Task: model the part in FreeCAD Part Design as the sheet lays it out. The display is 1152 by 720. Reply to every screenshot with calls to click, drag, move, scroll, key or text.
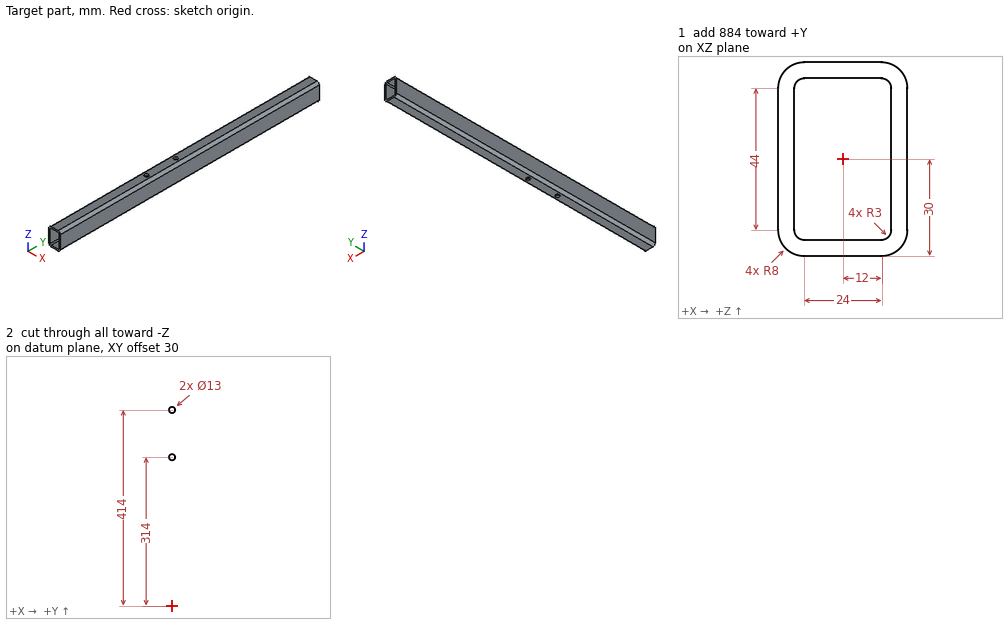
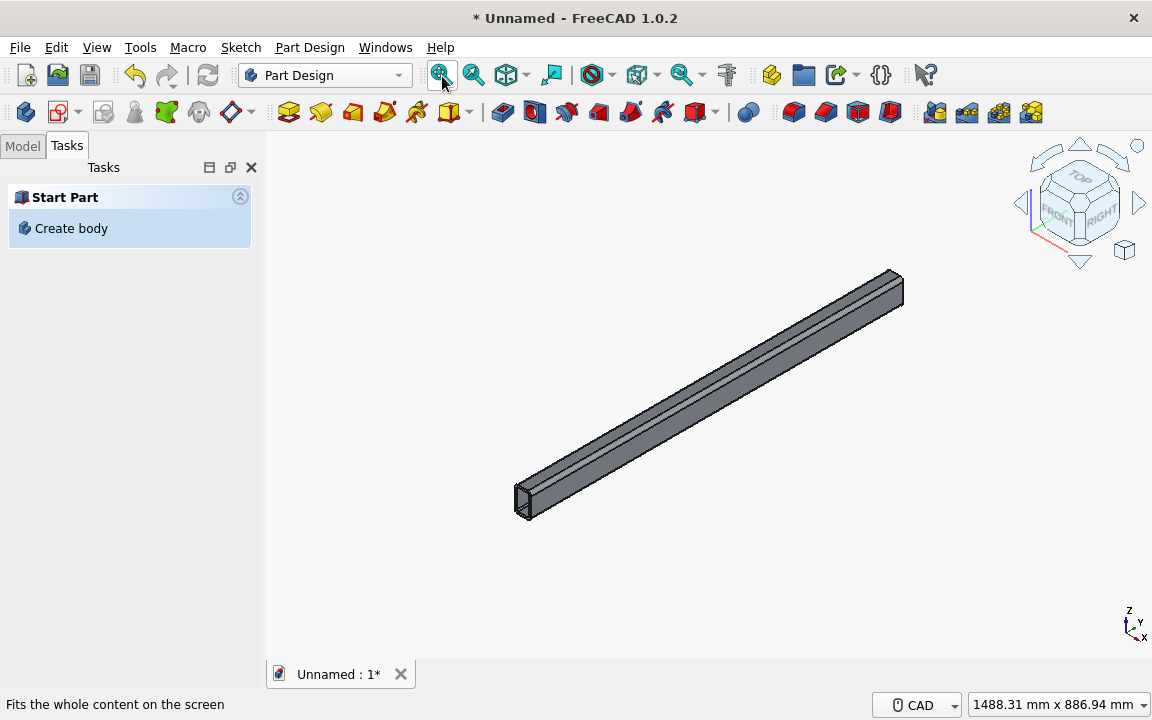
key(2)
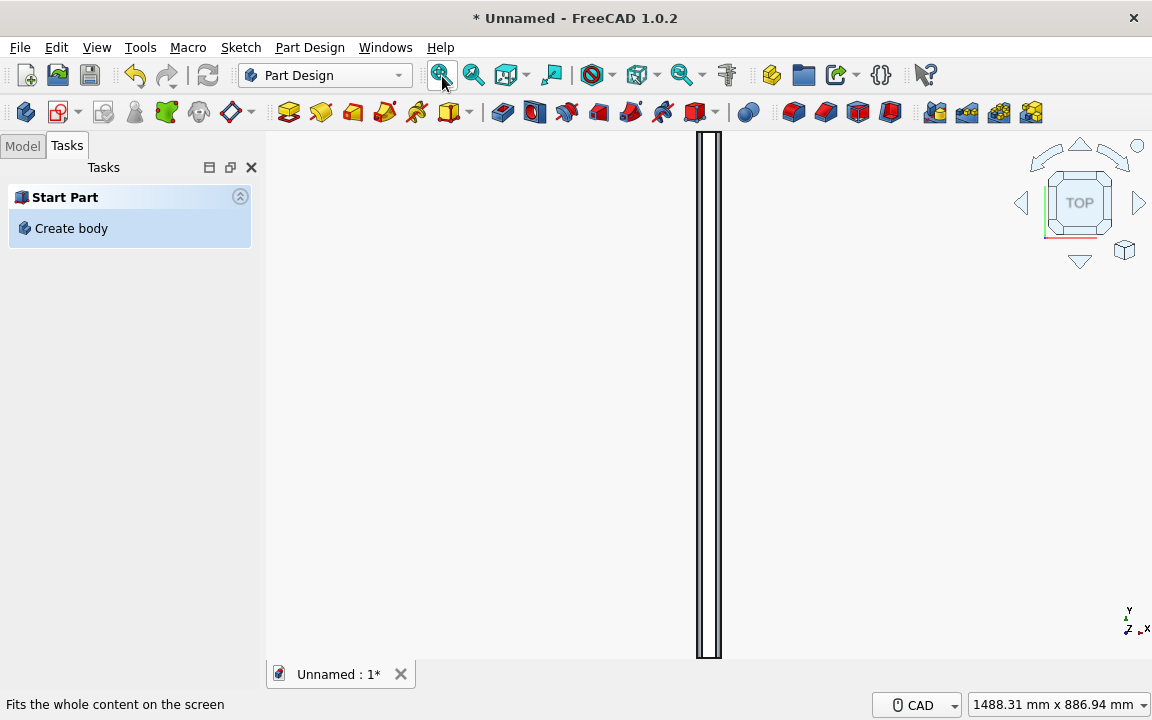
key(4)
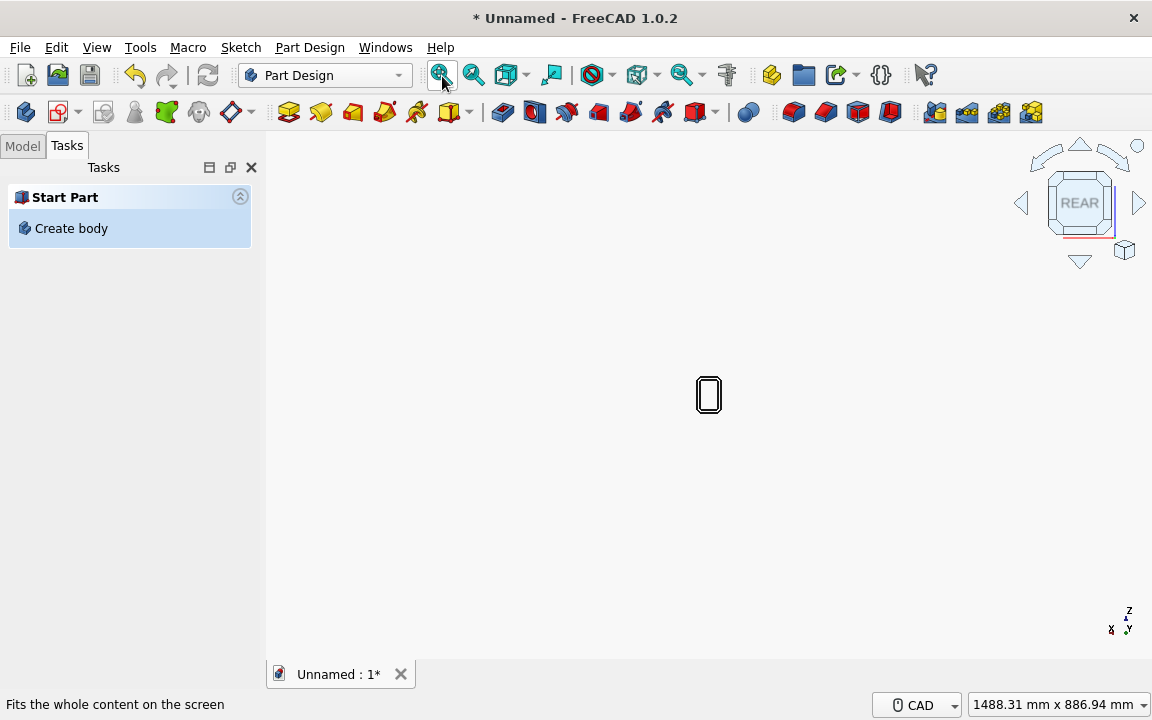
key(v)
key(f)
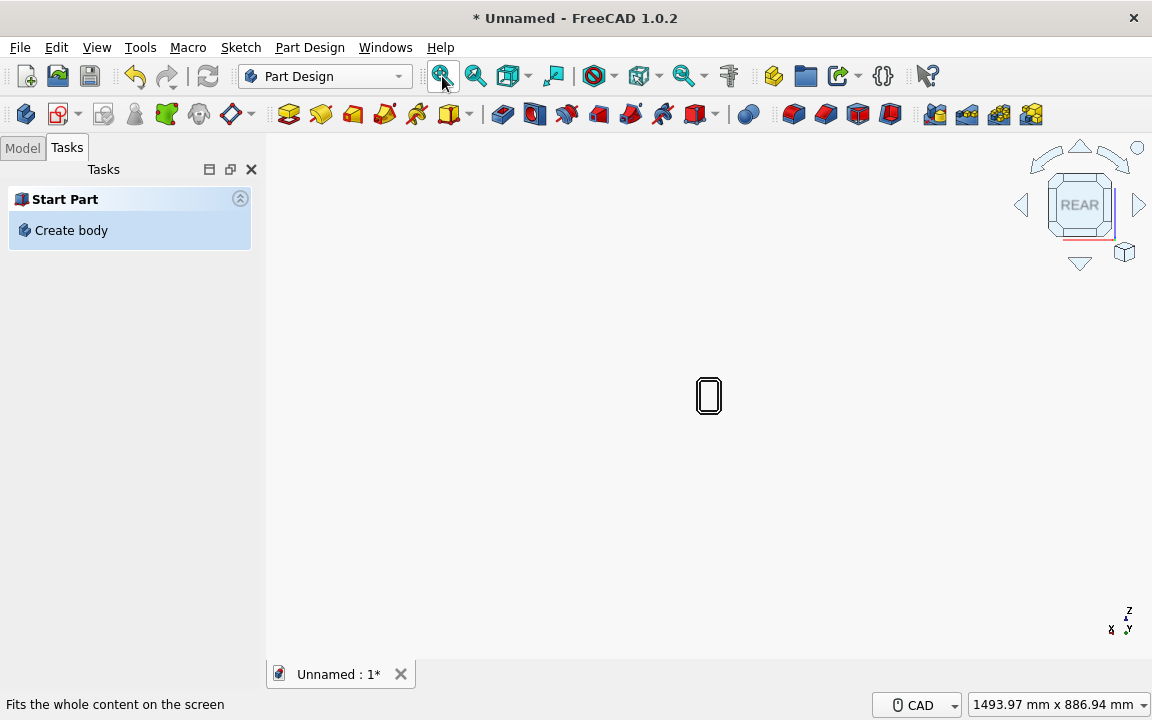
click(23, 147)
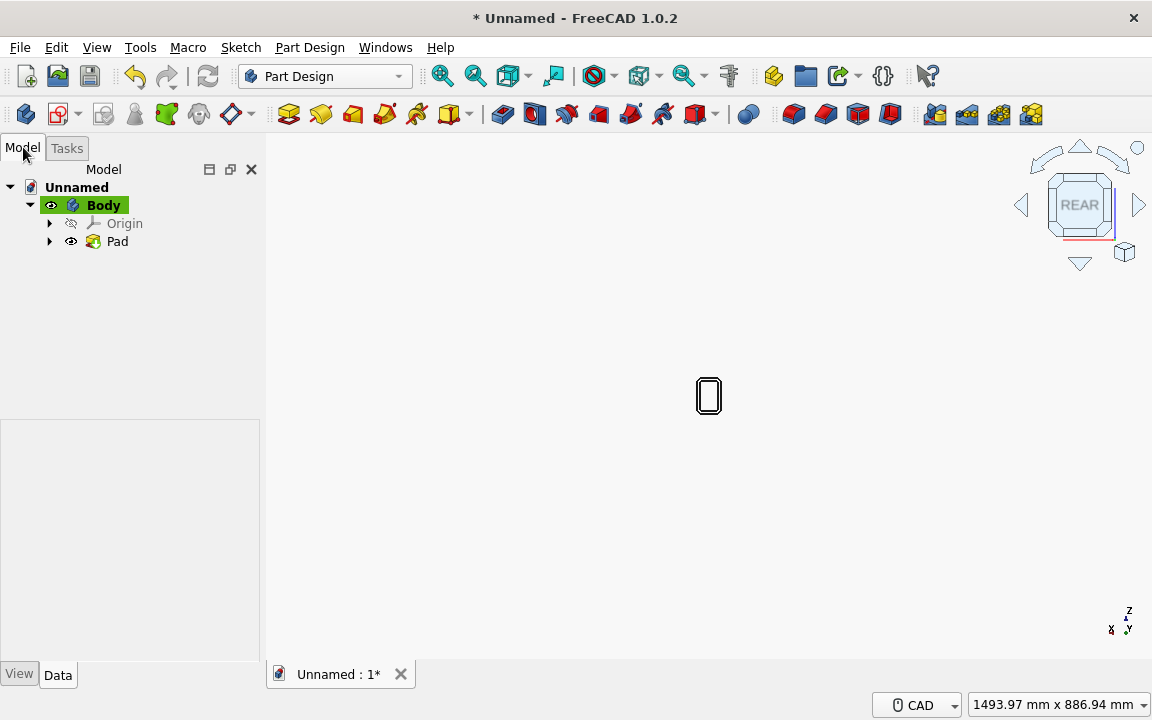
click(50, 223)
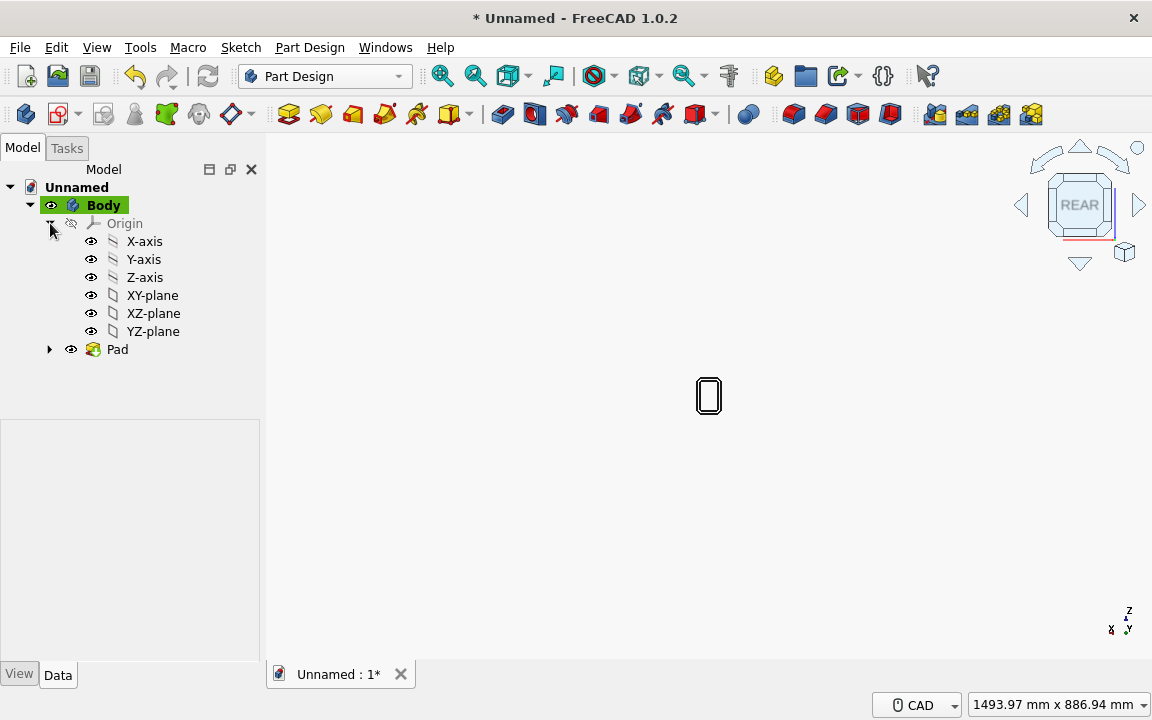
click(136, 295)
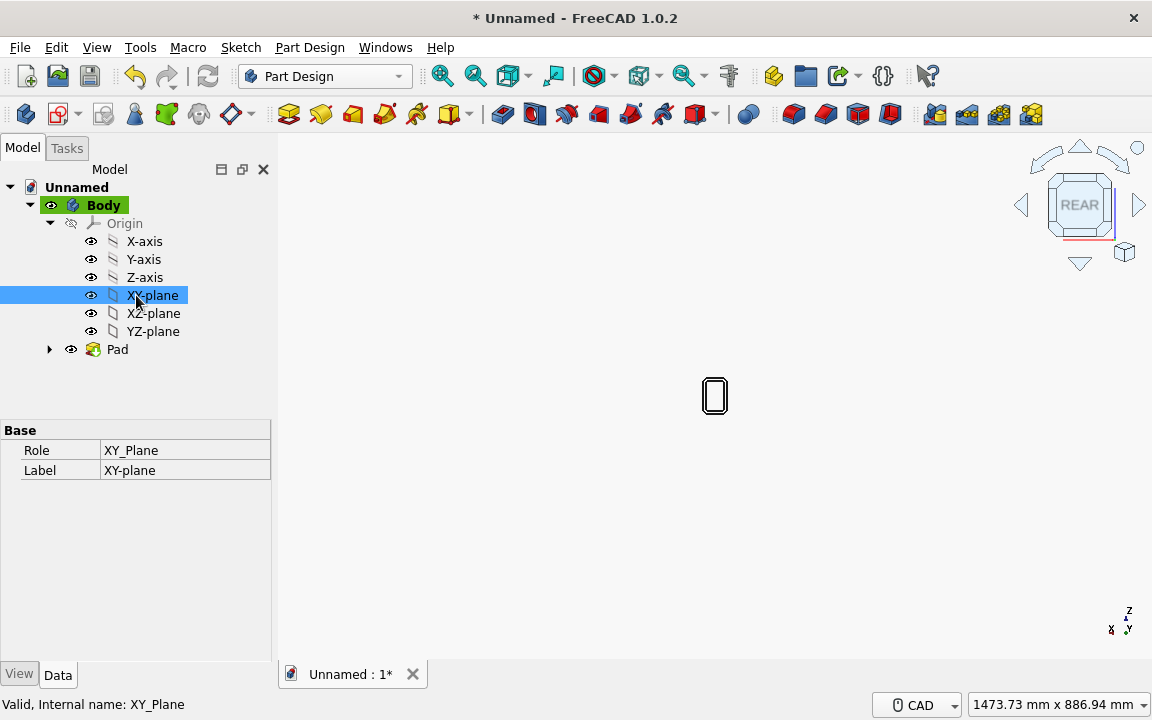
click(232, 114)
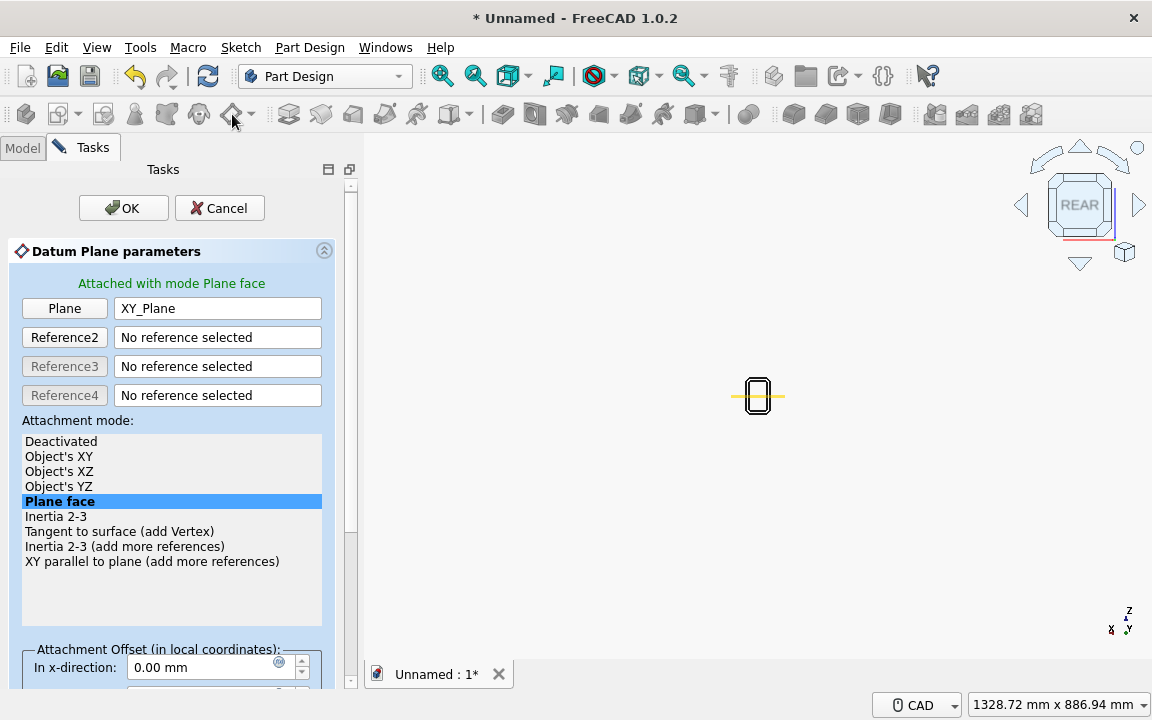
scroll(351, 434, down, 2)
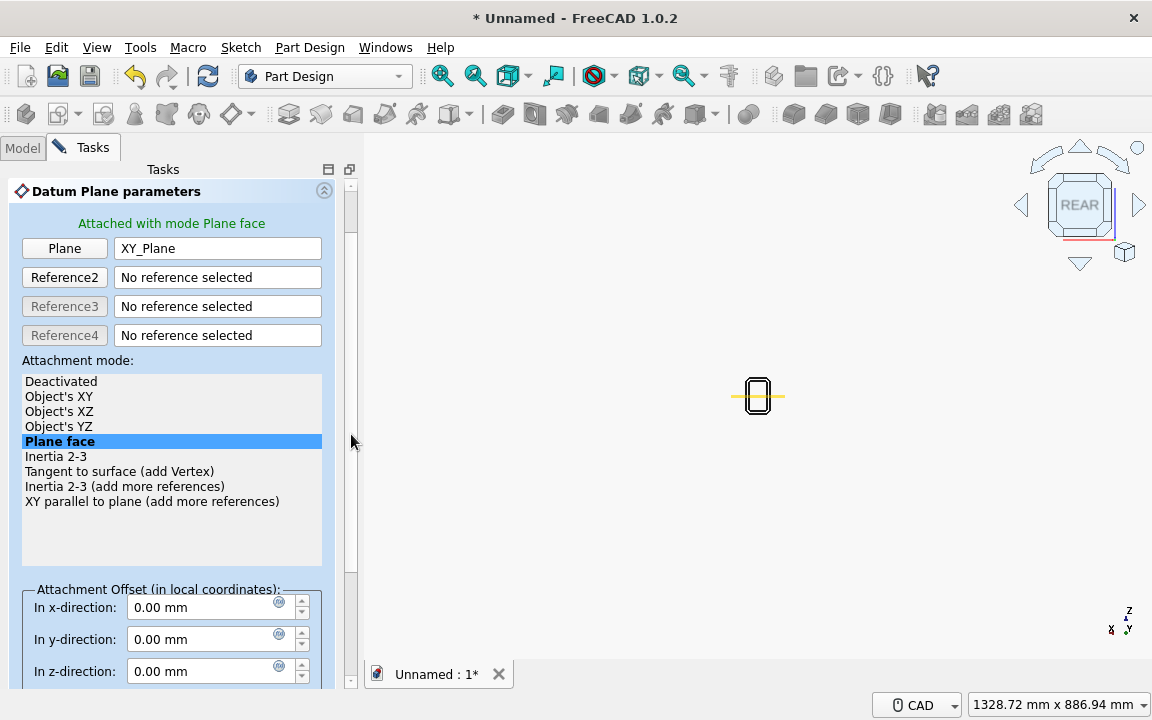
triple_click(210, 611)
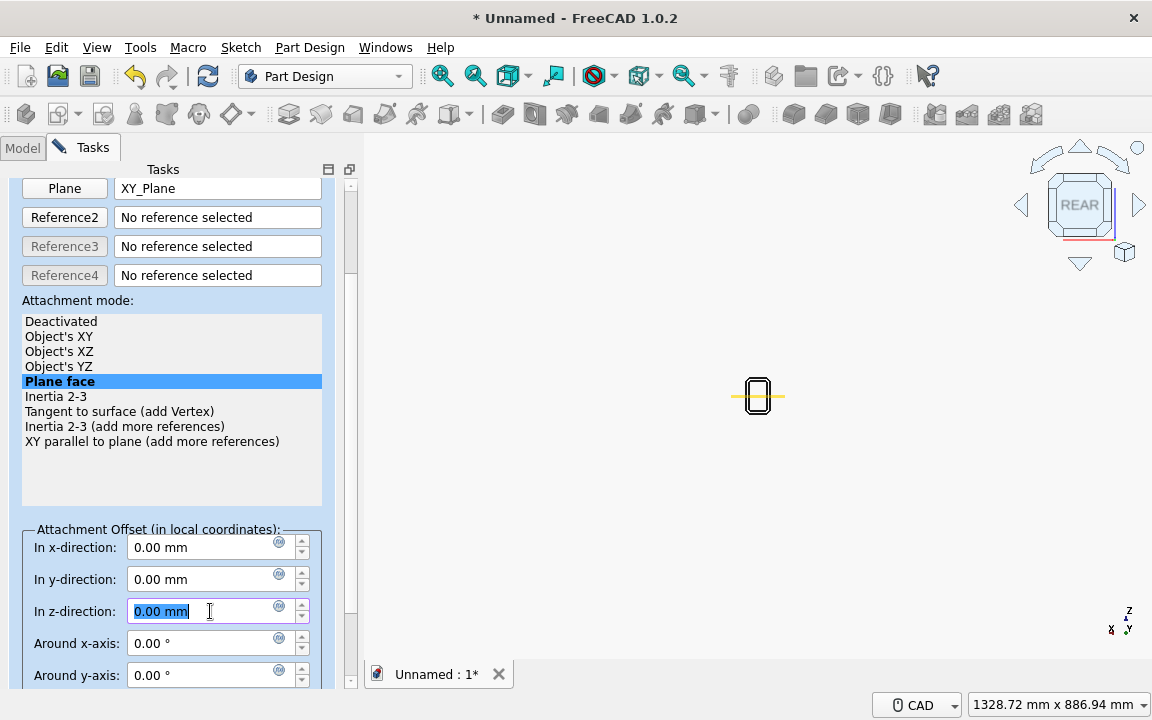
text(30)
key(Tab)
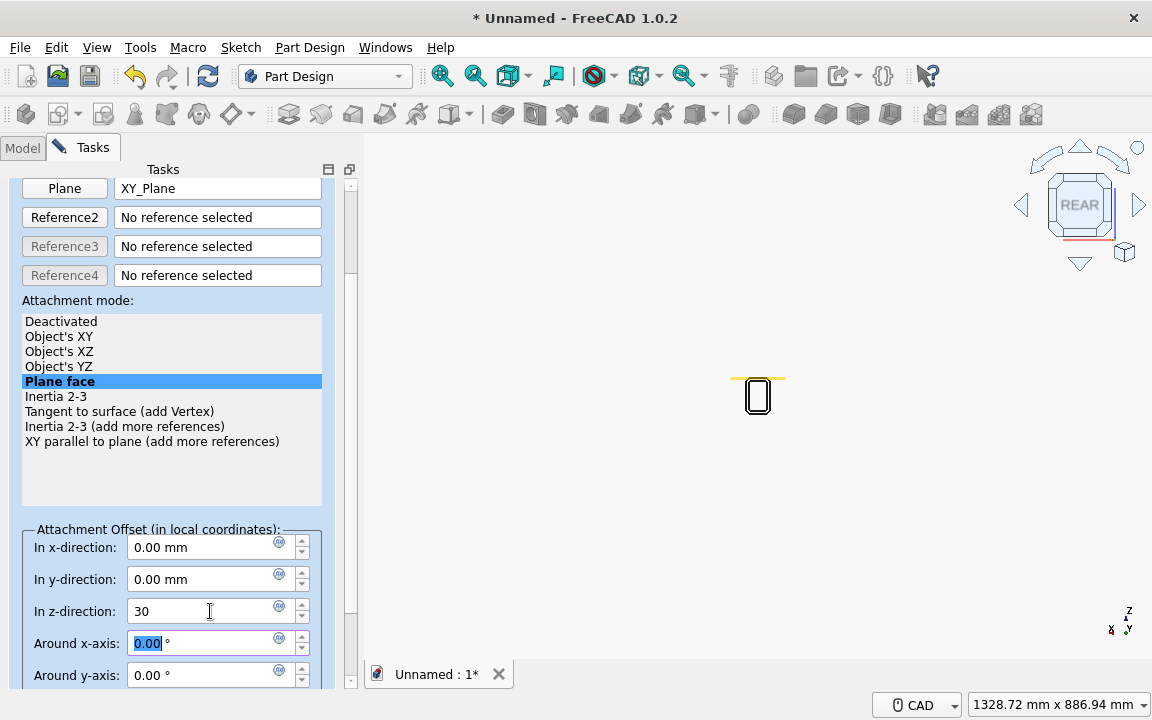
scroll(351, 434, up, 3)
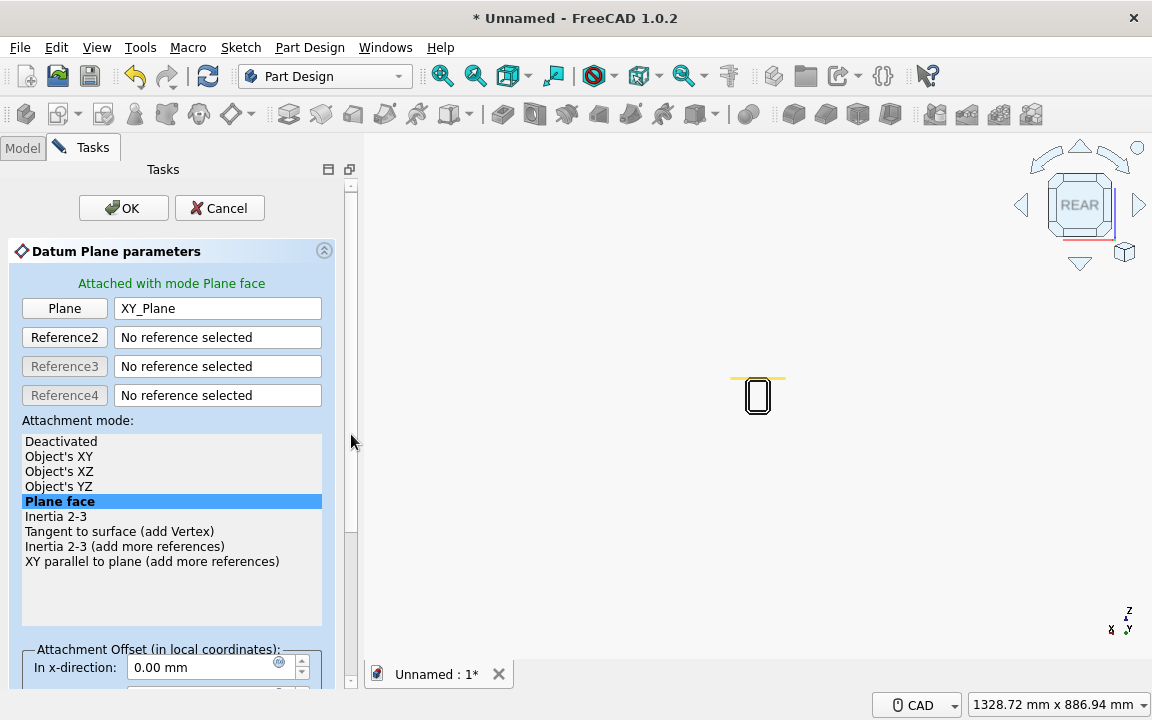
click(124, 208)